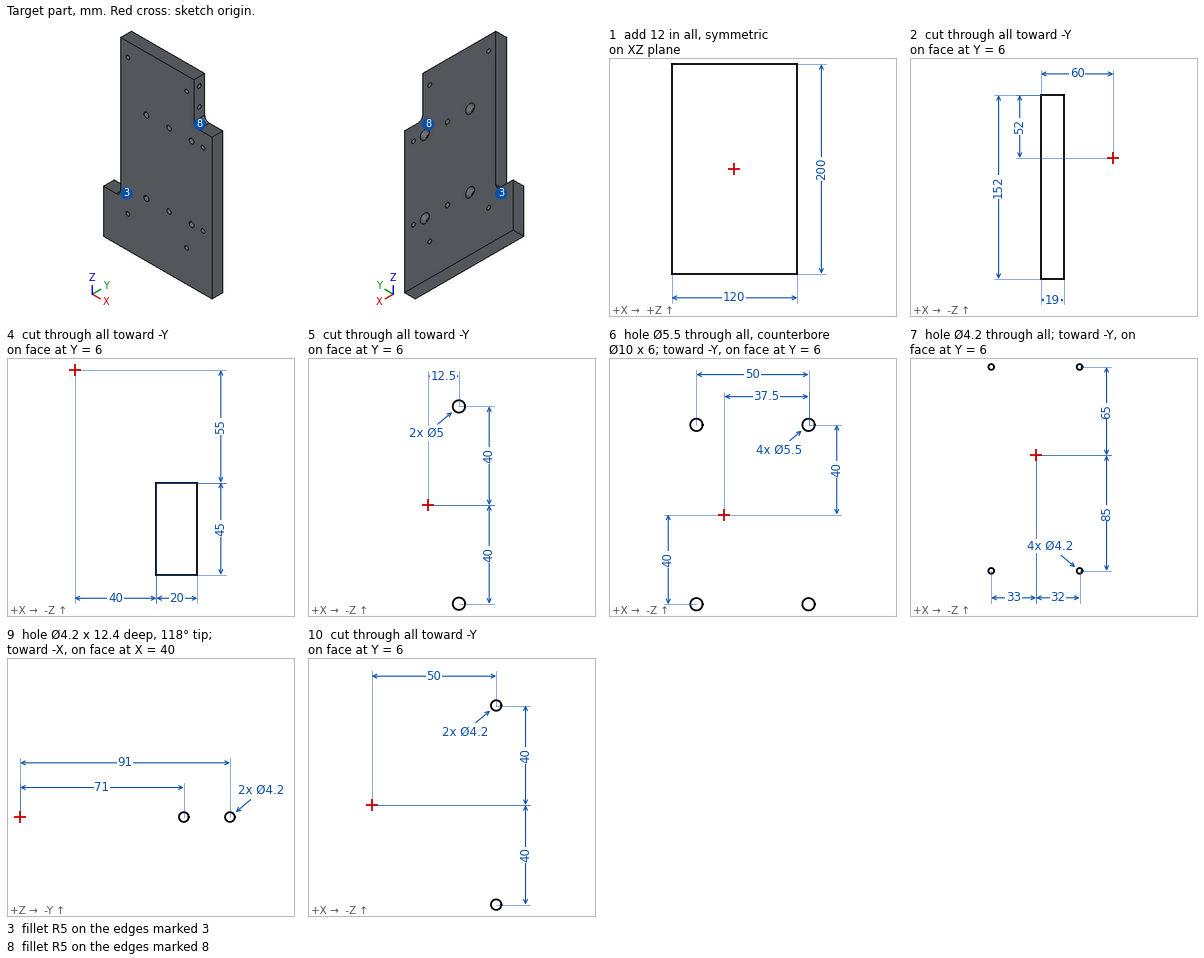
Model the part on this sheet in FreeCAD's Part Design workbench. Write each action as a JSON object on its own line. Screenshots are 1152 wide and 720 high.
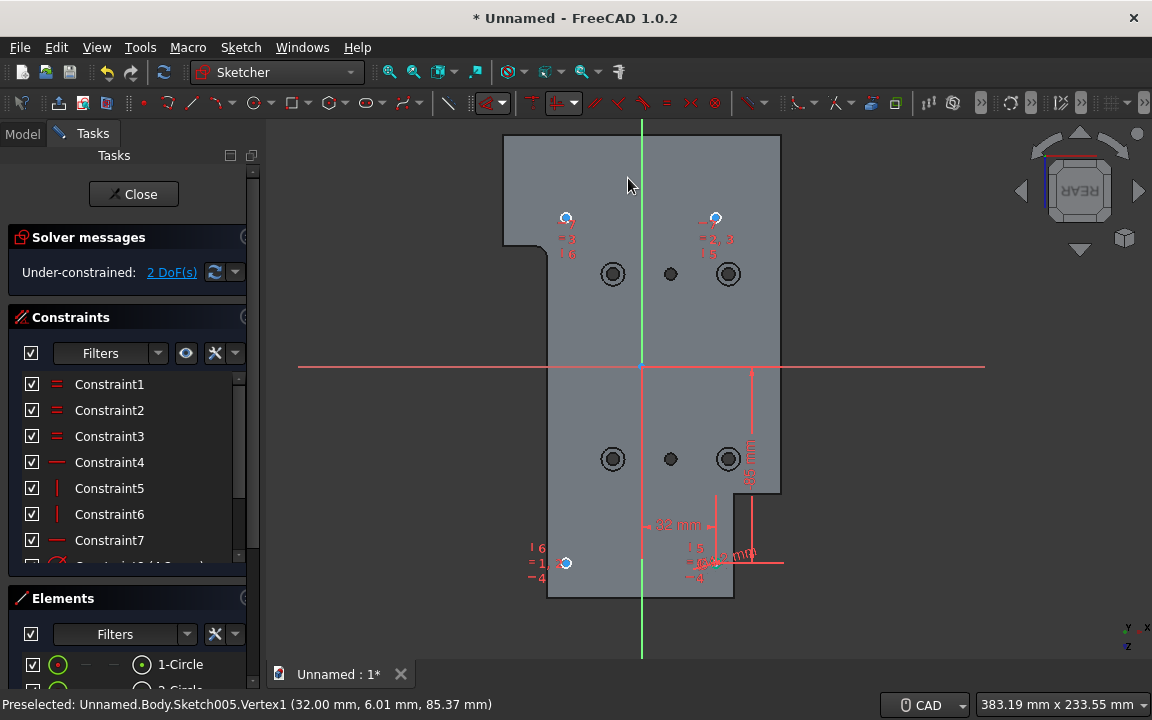
{"action": "left_click", "coordinate": [566, 563]}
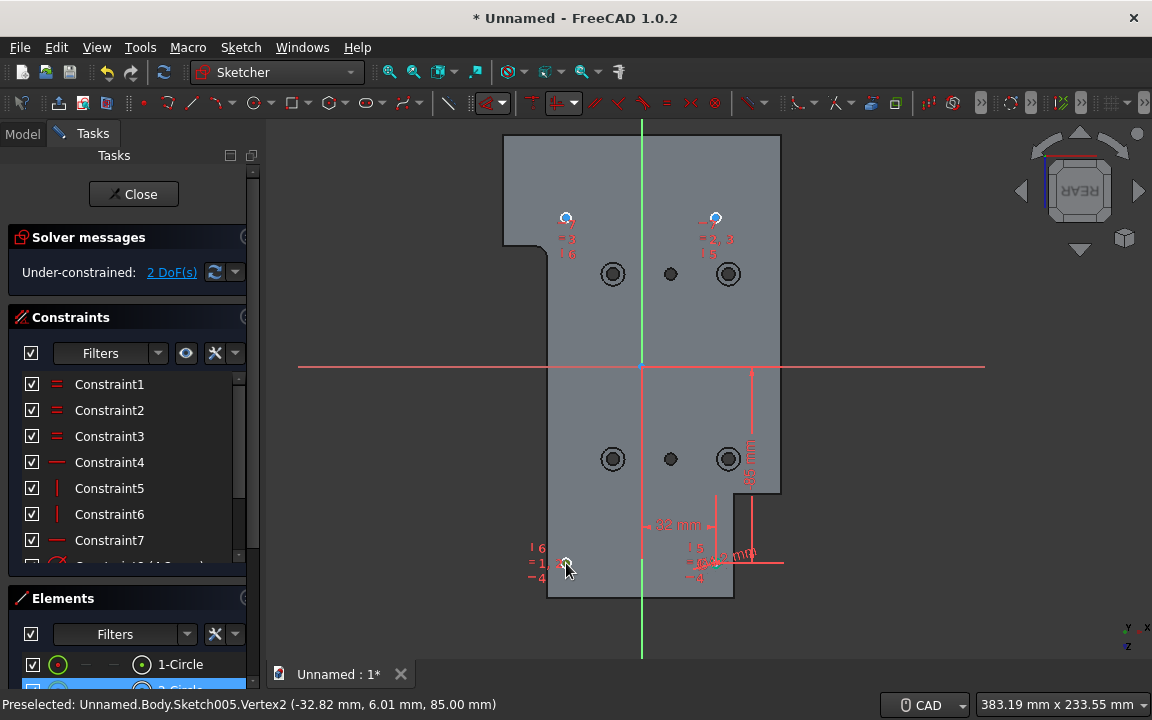
{"action": "left_click", "coordinate": [504, 104]}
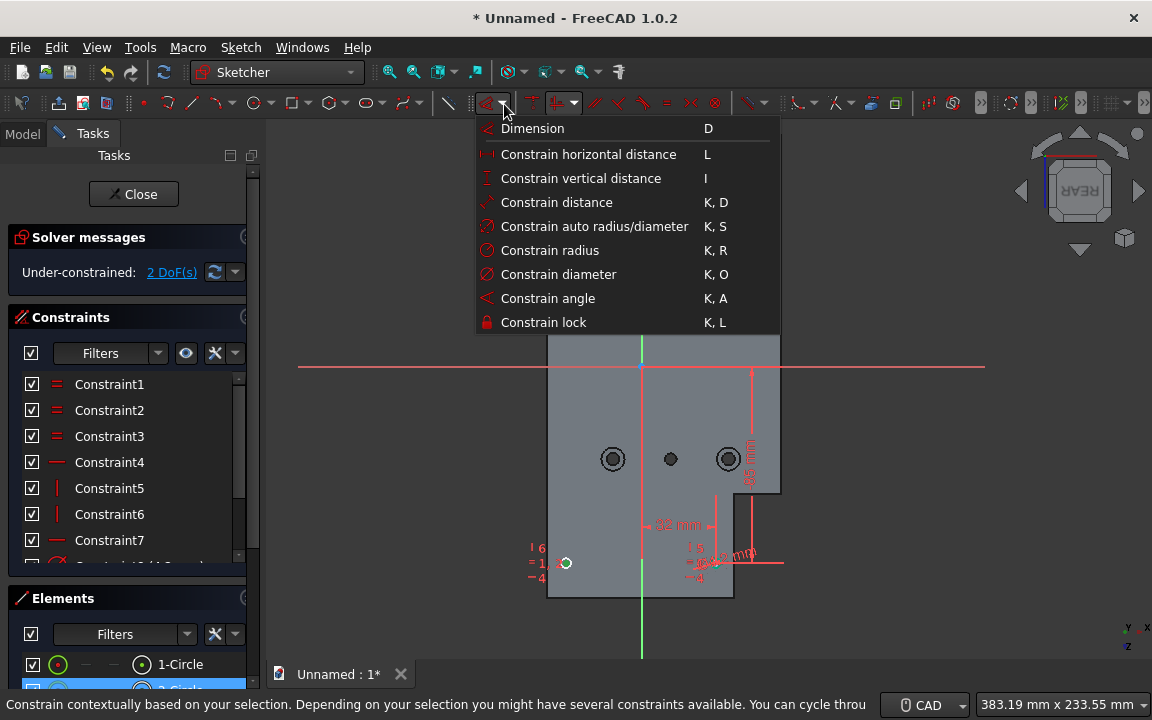
{"action": "left_click", "coordinate": [628, 154]}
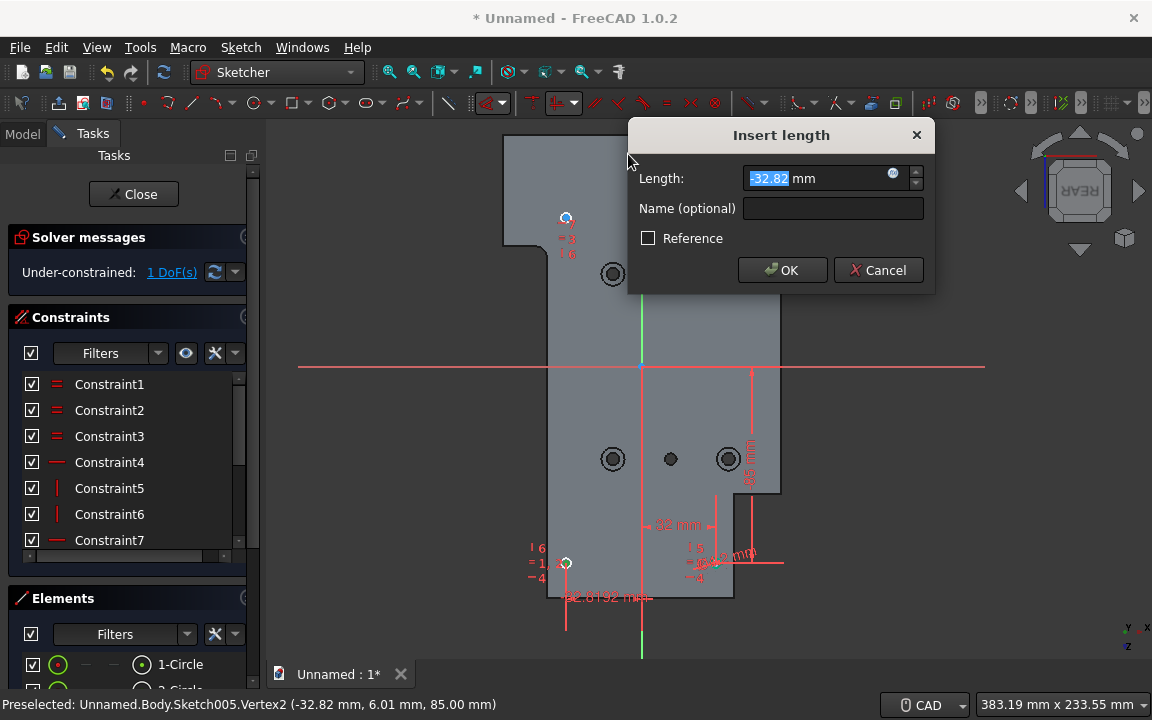
{"action": "type", "text": "-33"}
{"action": "key", "text": "Return"}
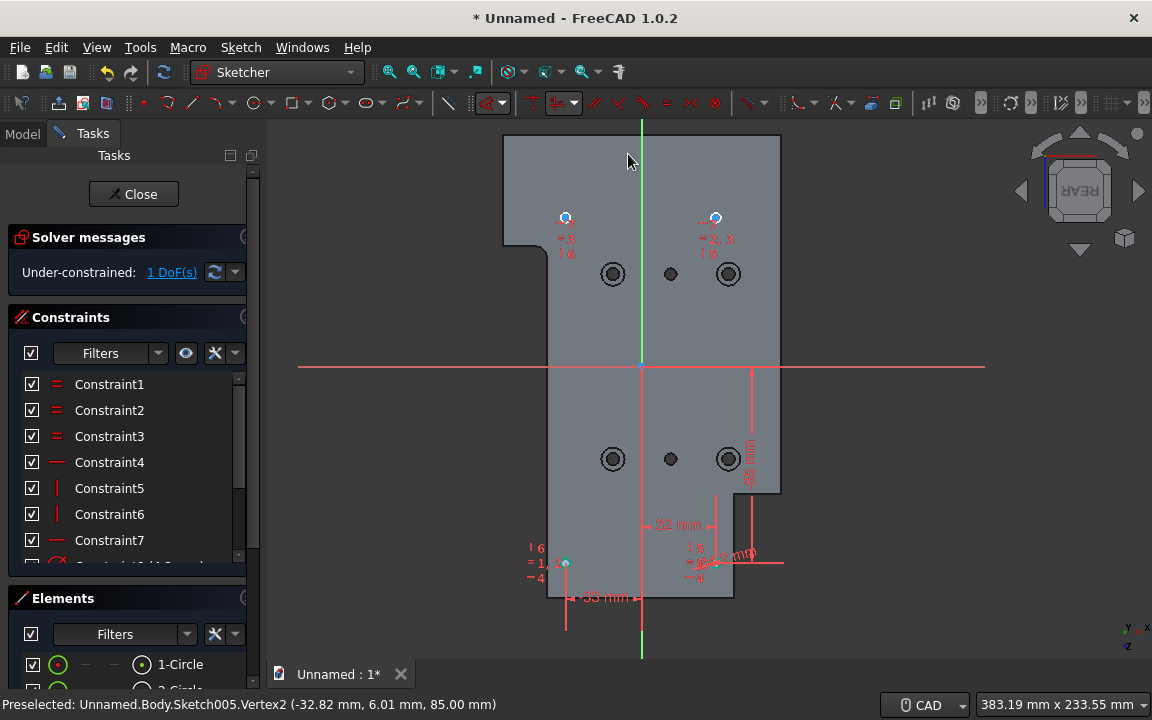
{"action": "left_click", "coordinate": [716, 218]}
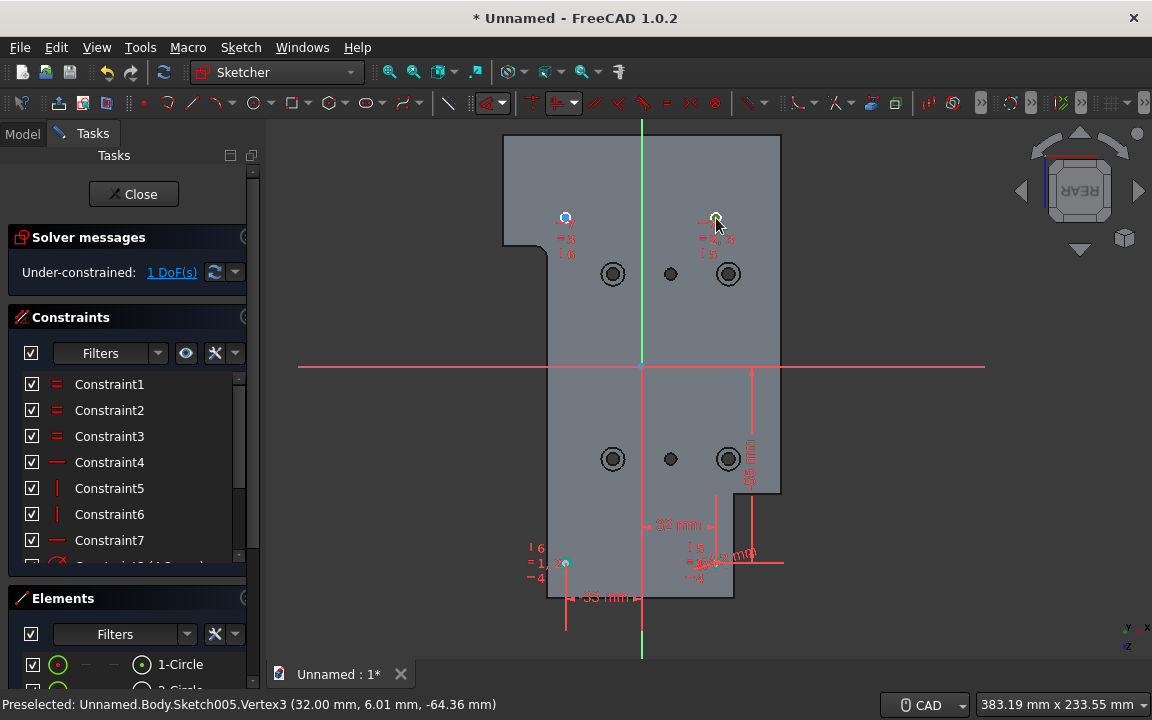
{"action": "left_click", "coordinate": [504, 104]}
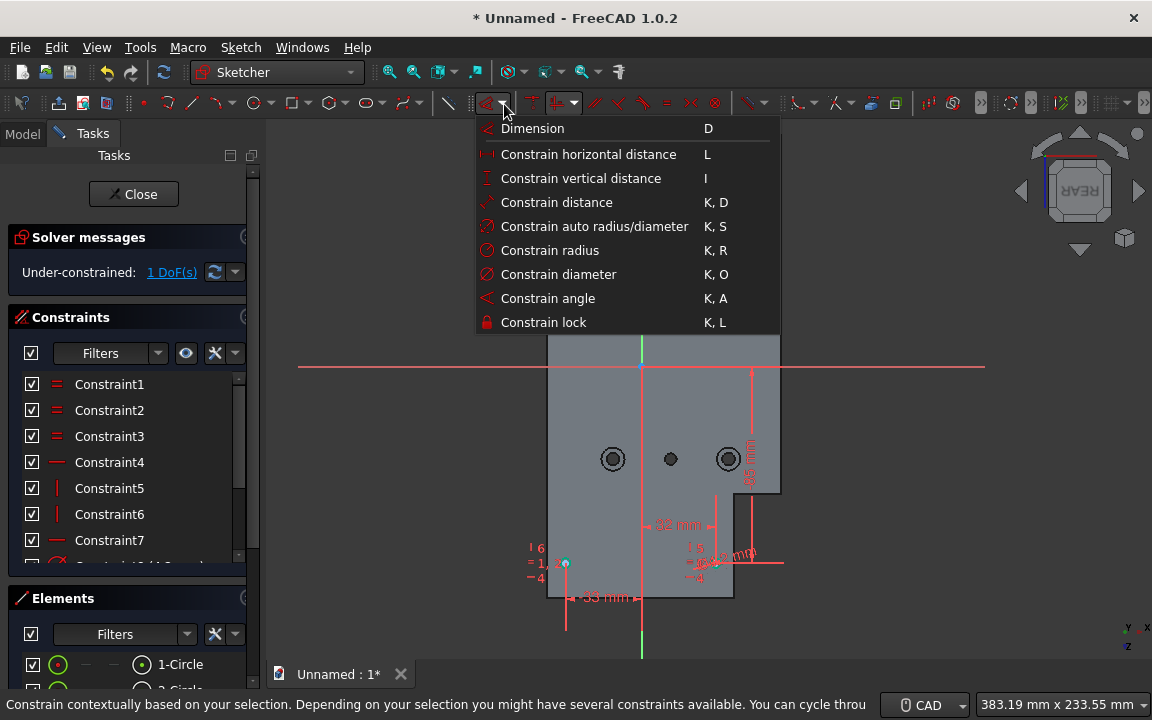
{"action": "left_click", "coordinate": [628, 178]}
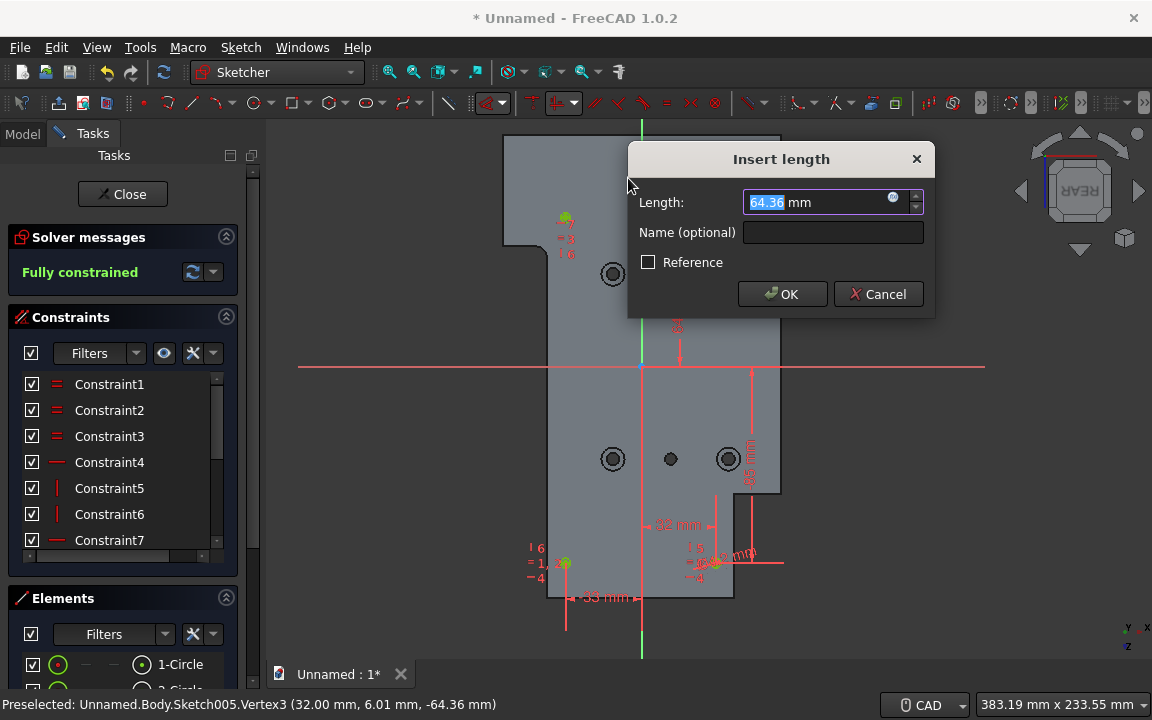
{"action": "type", "text": "65"}
{"action": "key", "text": "Return"}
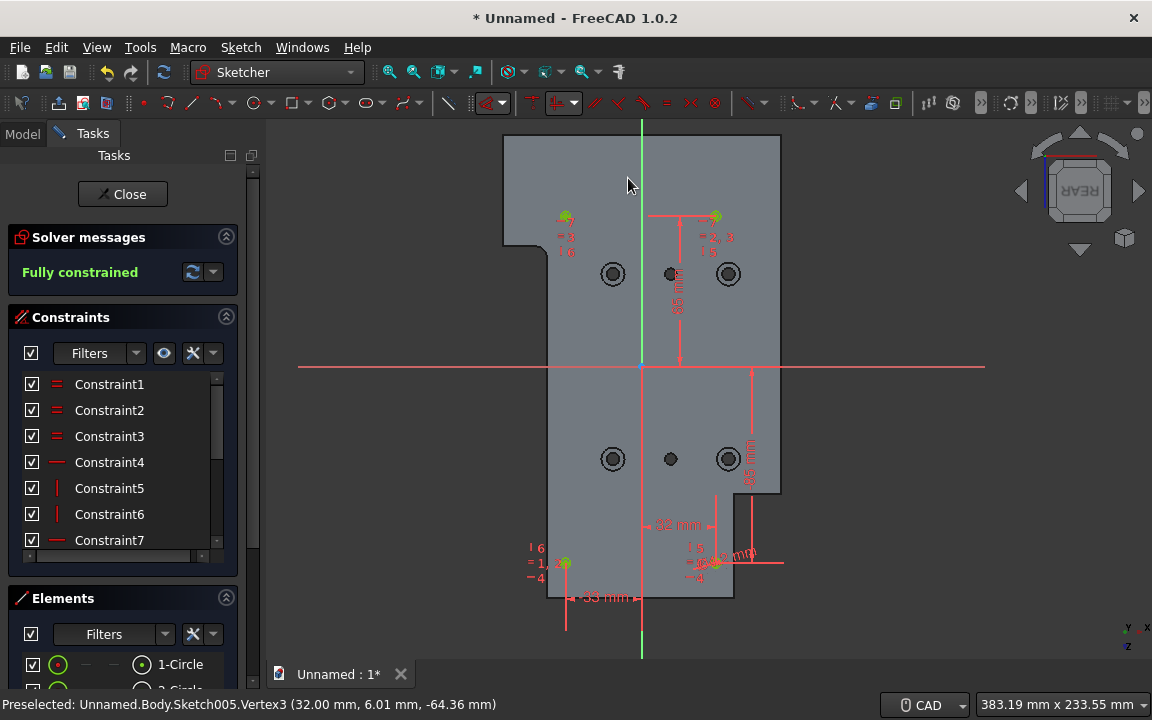
{"action": "left_click", "coordinate": [123, 194]}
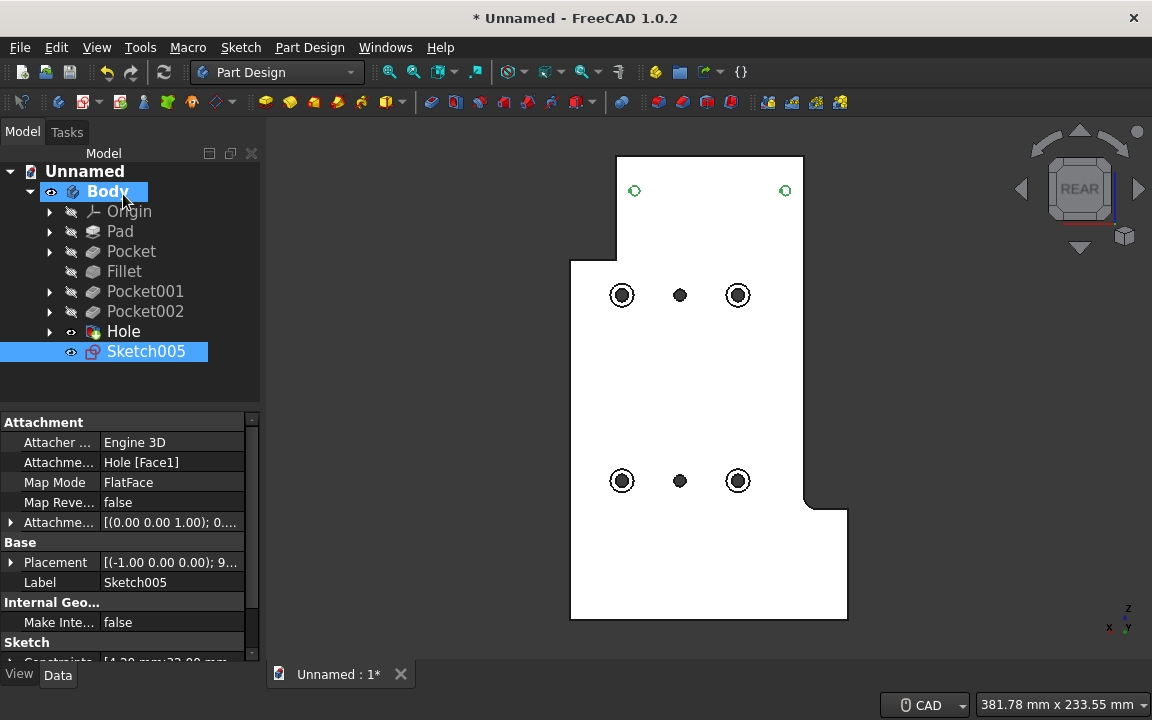
{"action": "left_click", "coordinate": [456, 102]}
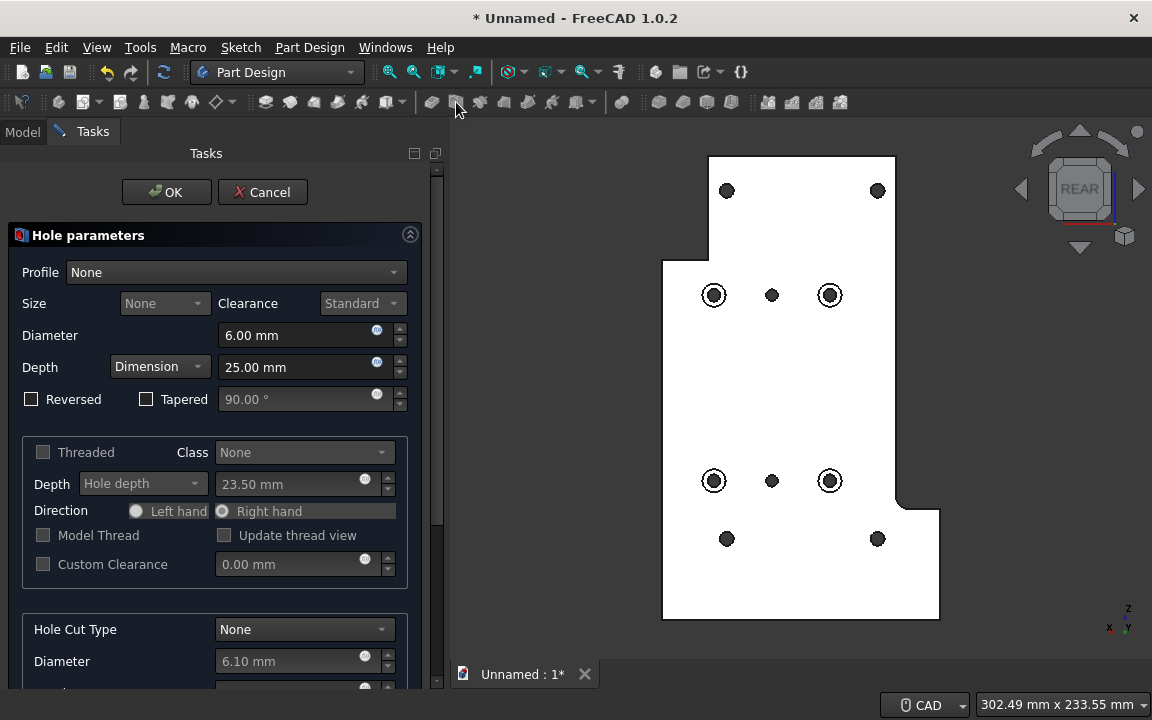
{"action": "triple_click", "coordinate": [305, 335]}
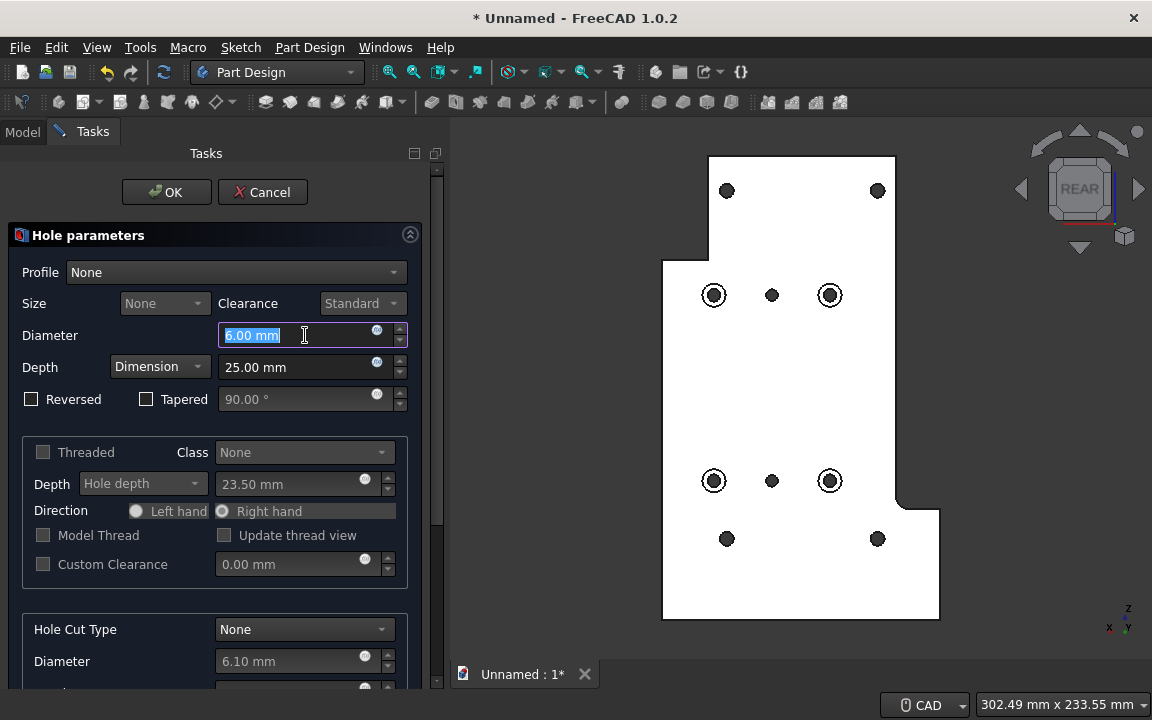
{"action": "type", "text": "4.2"}
{"action": "key", "text": "Tab"}